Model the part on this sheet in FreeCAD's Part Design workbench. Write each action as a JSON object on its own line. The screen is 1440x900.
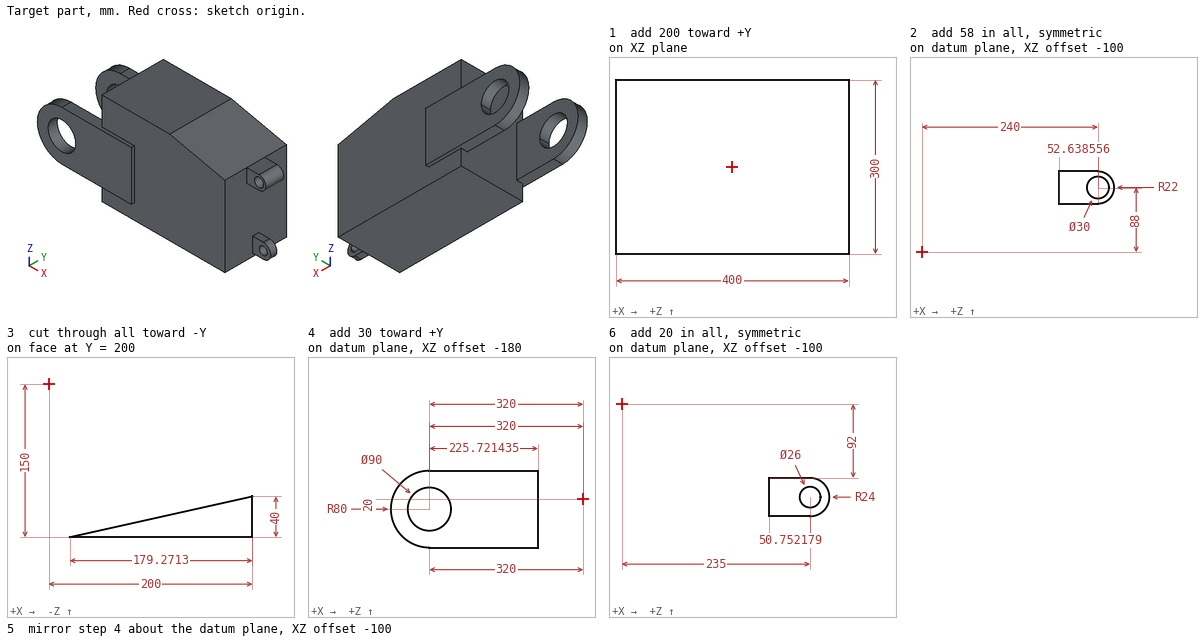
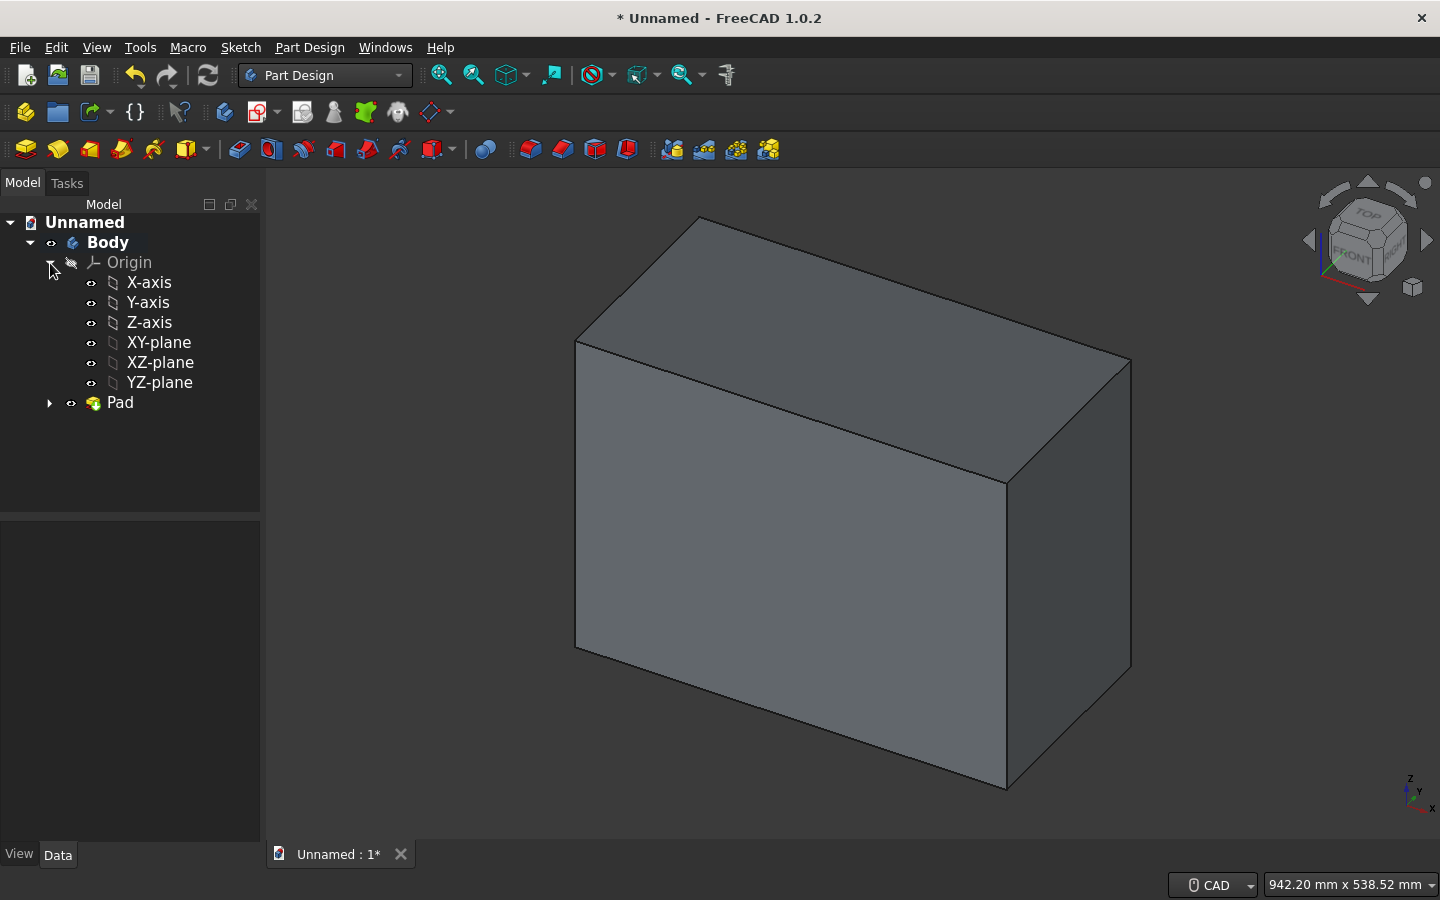
{"action": "left_click", "coordinate": [136, 363]}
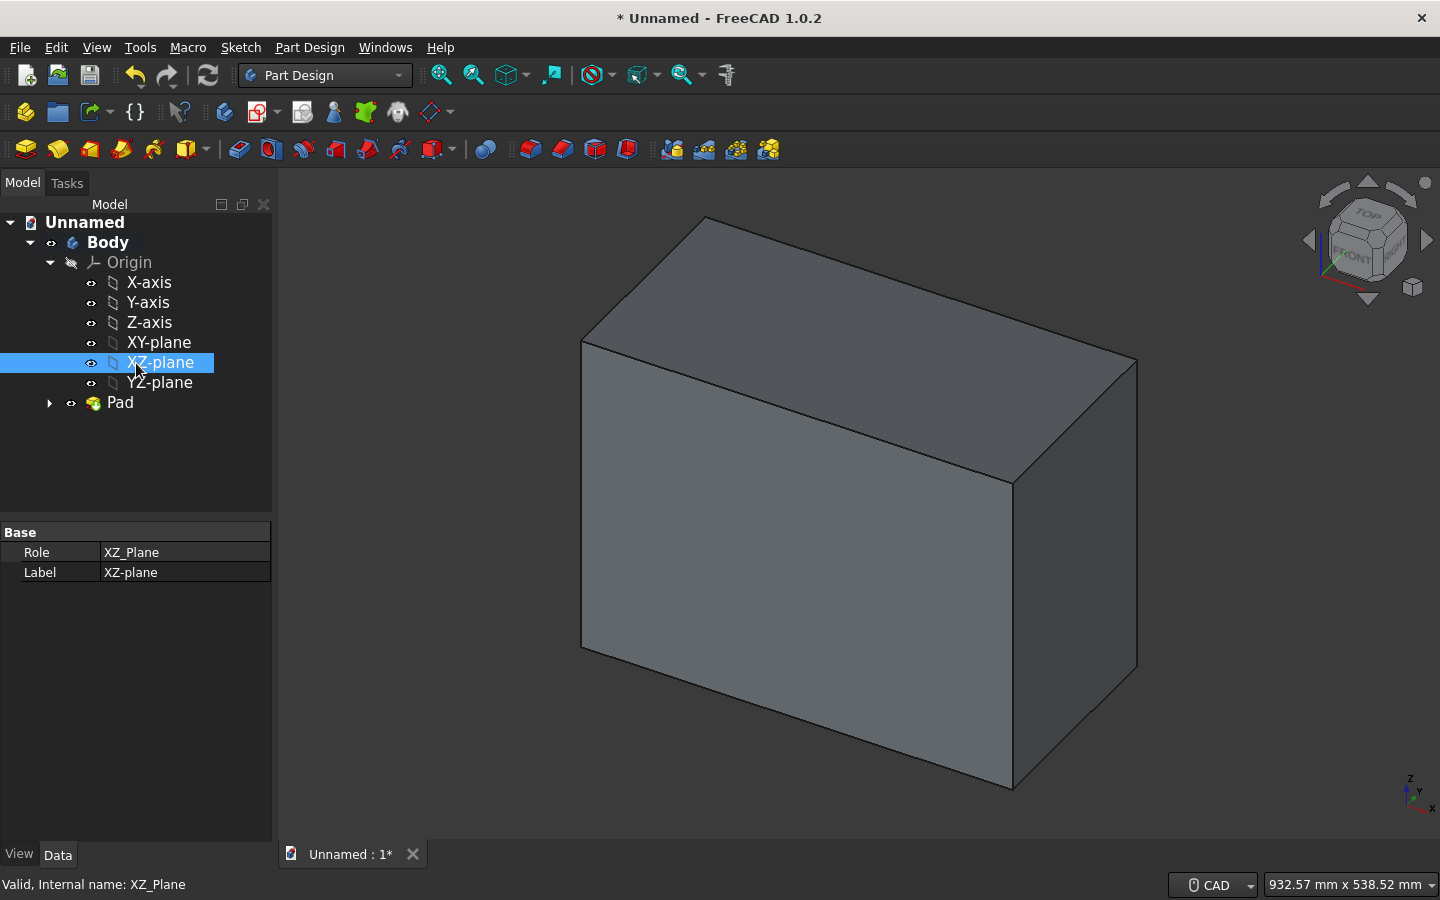
{"action": "left_click", "coordinate": [430, 112]}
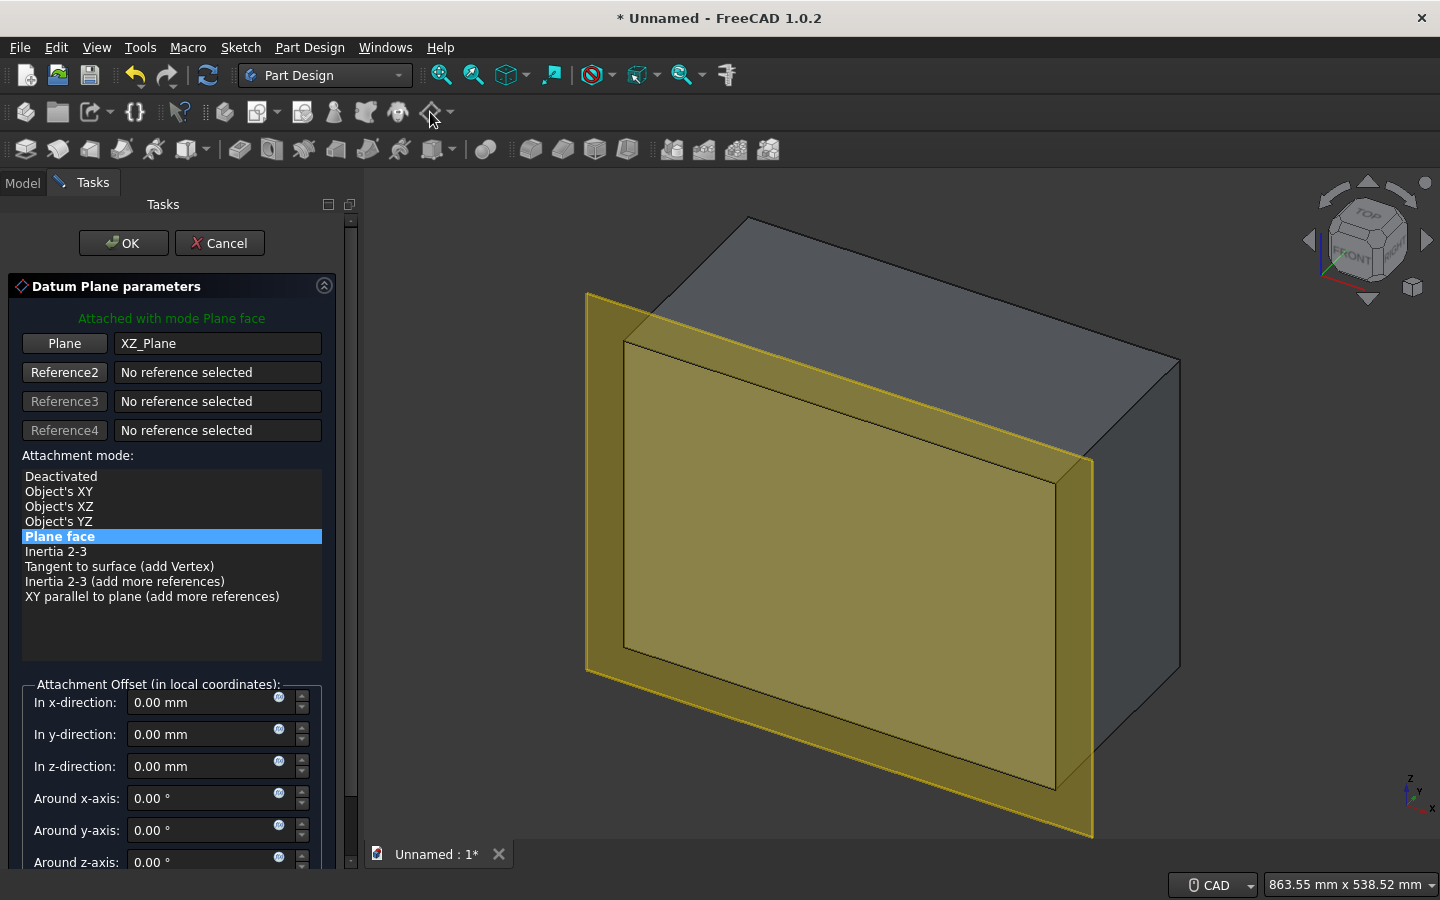
{"action": "triple_click", "coordinate": [210, 766]}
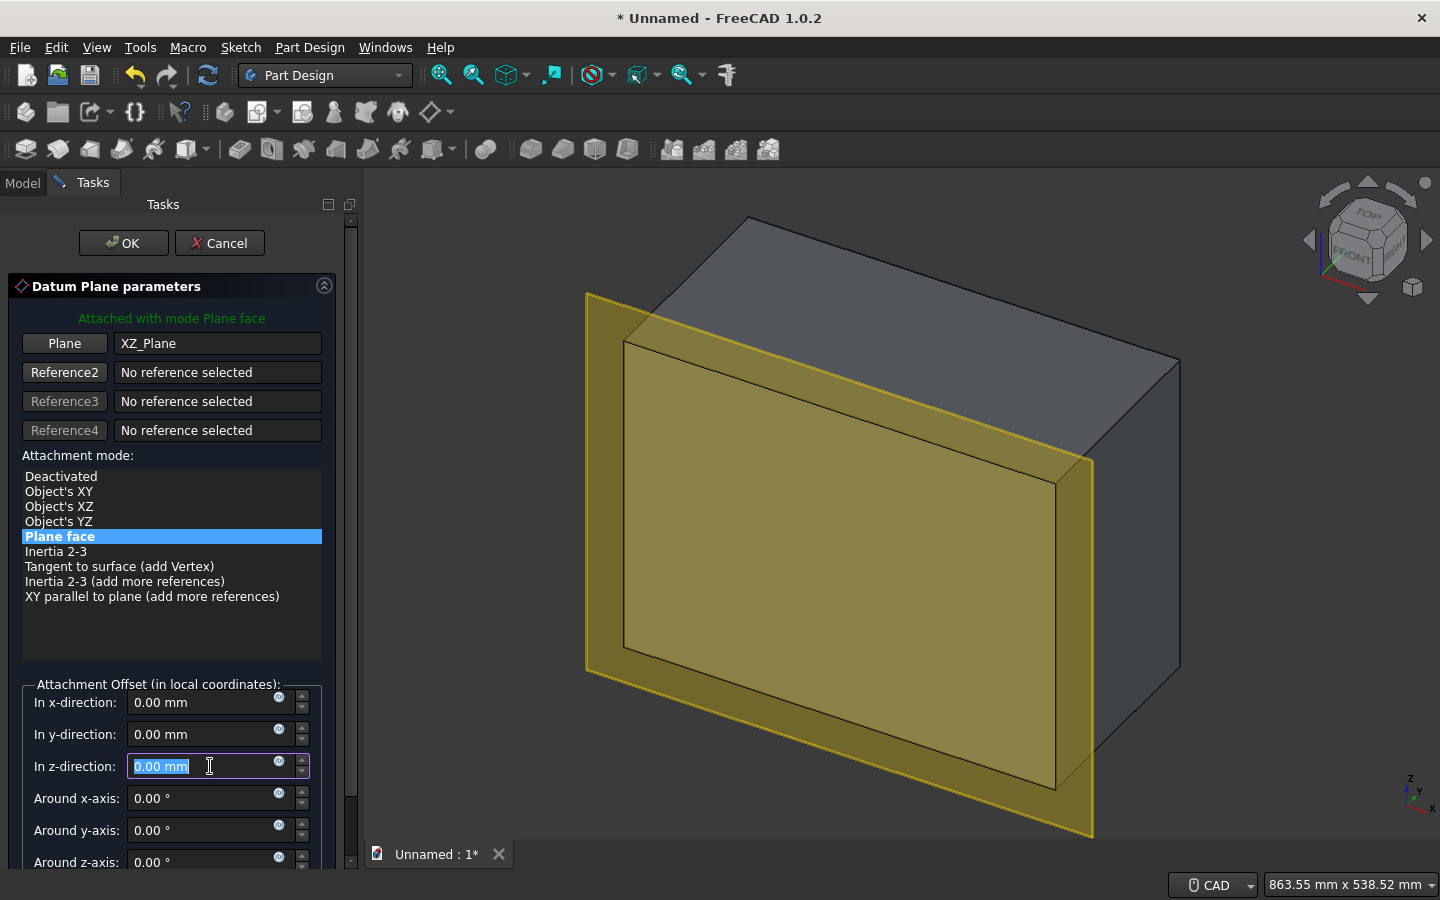
{"action": "type", "text": "-100"}
{"action": "key", "text": "Tab"}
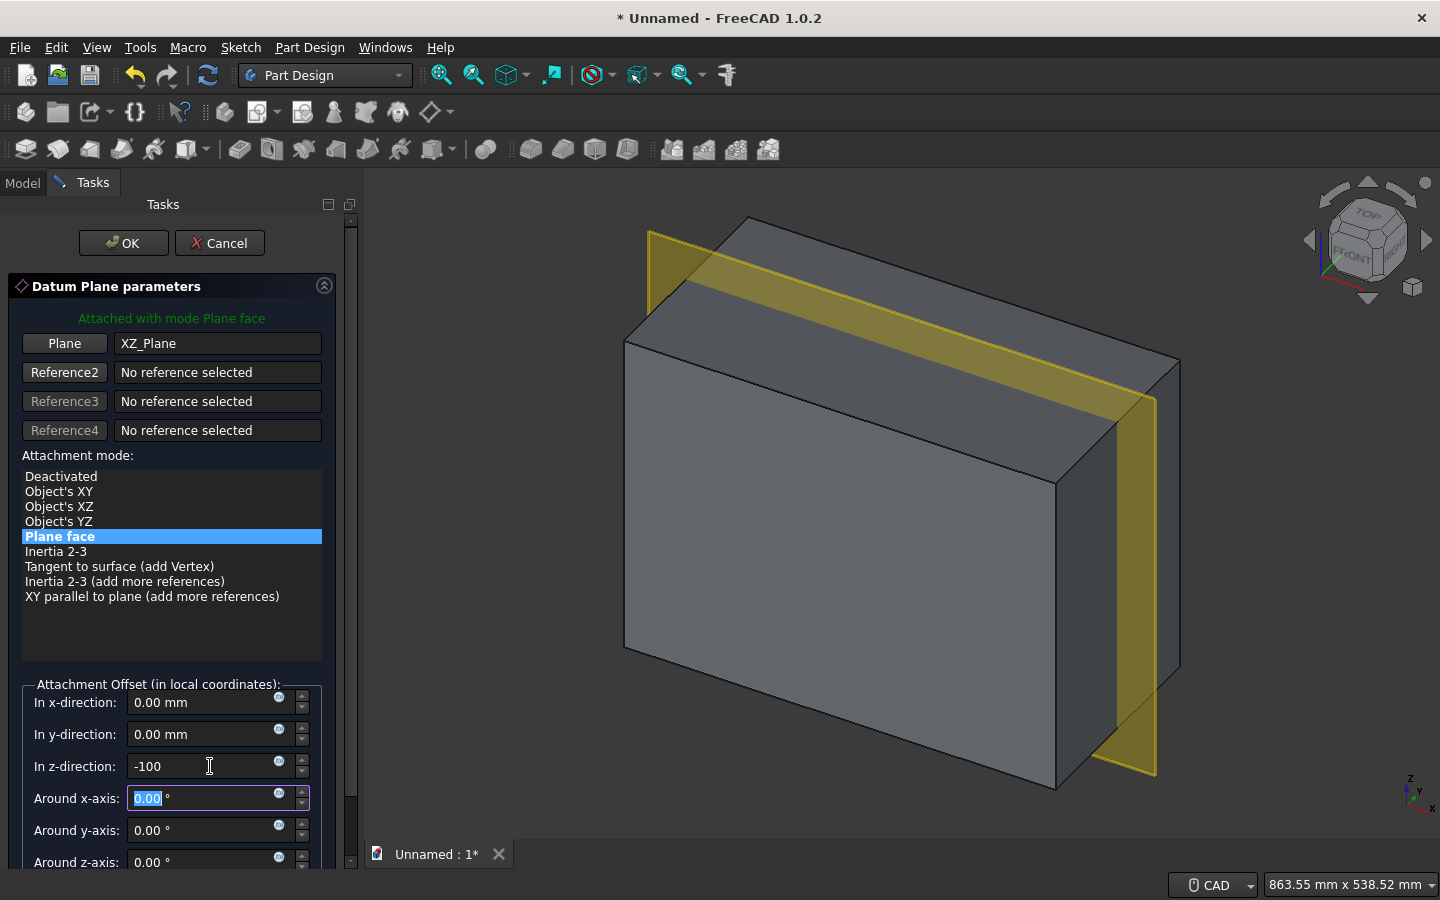
{"action": "left_click", "coordinate": [124, 243]}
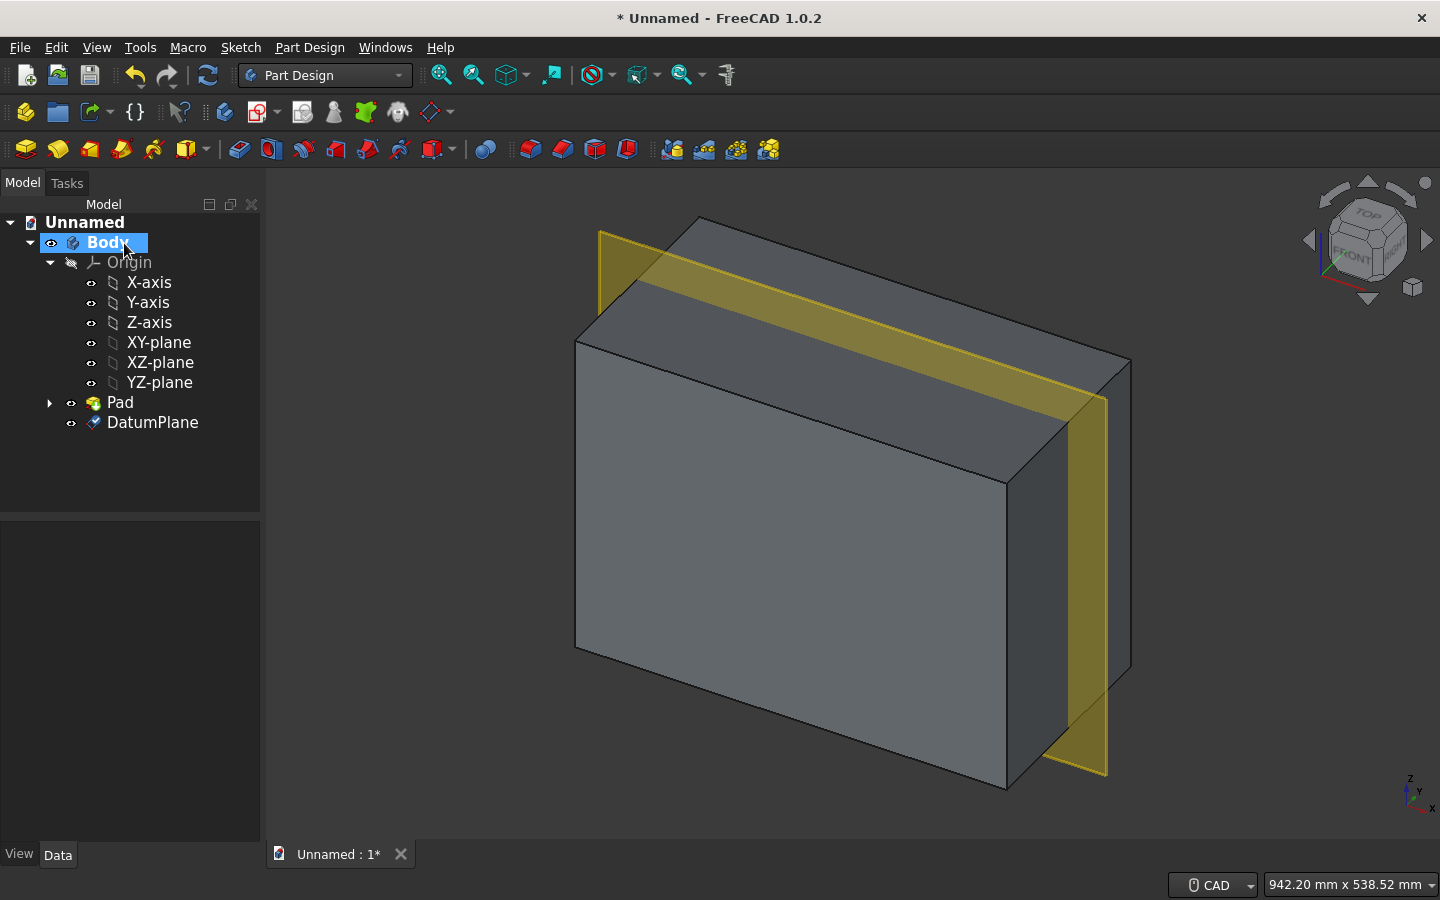
{"action": "left_click", "coordinate": [116, 423]}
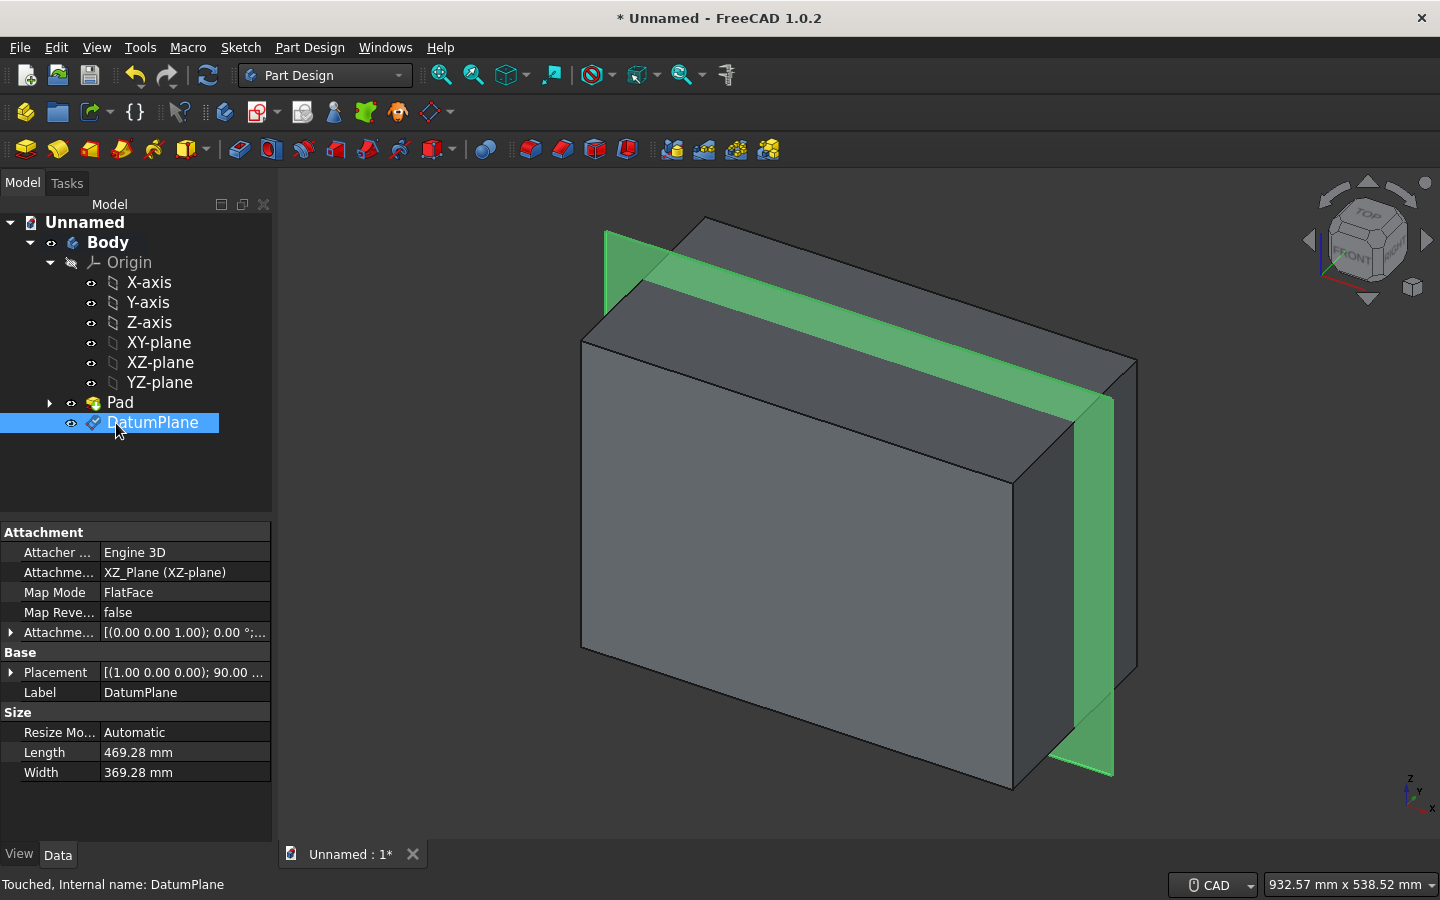
{"action": "left_click", "coordinate": [258, 112]}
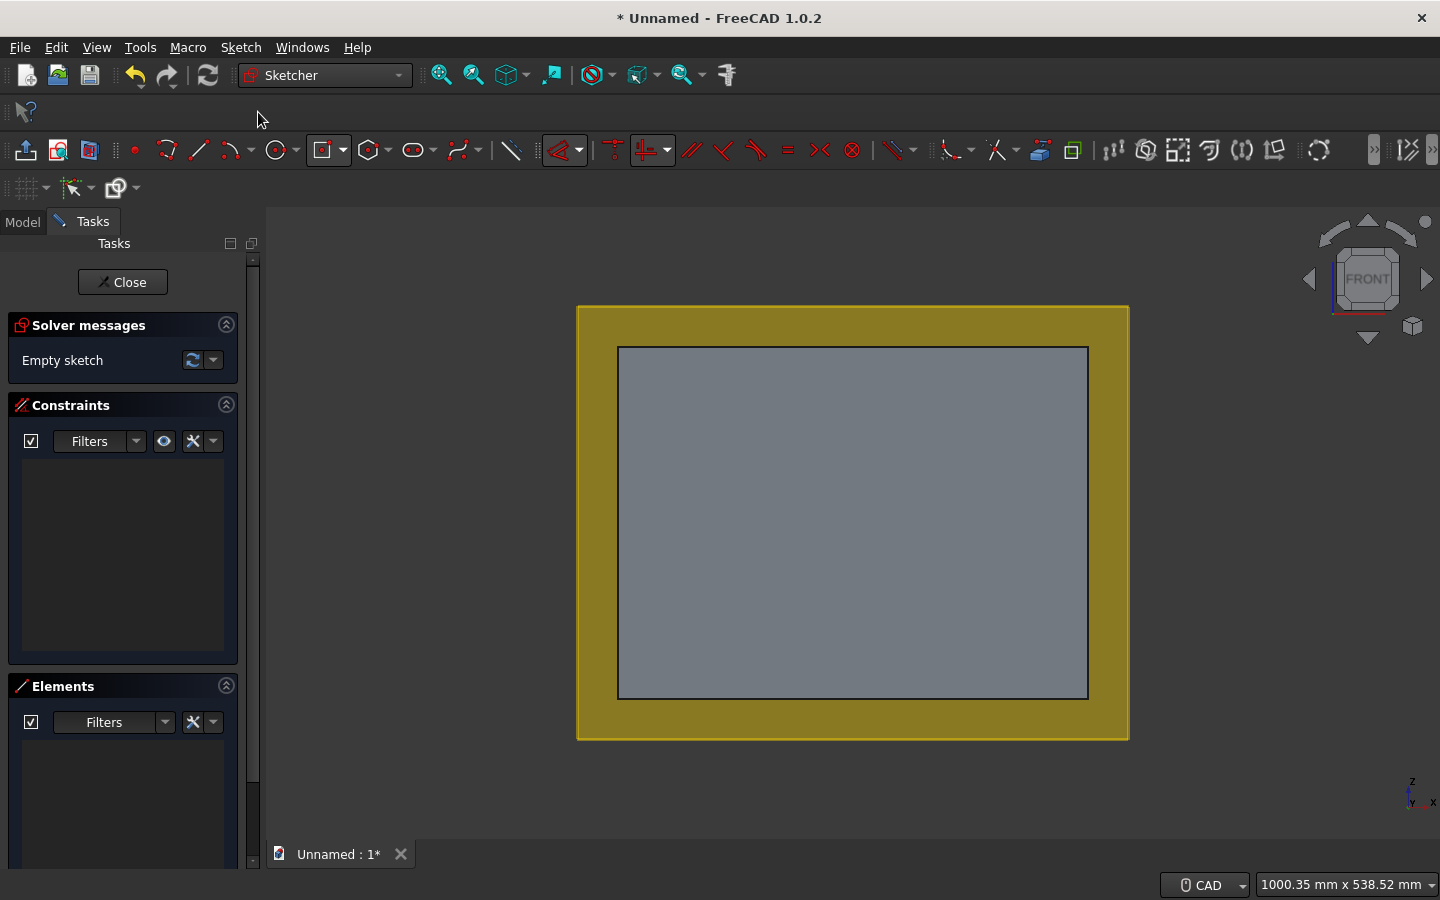
{"action": "left_click", "coordinate": [90, 150]}